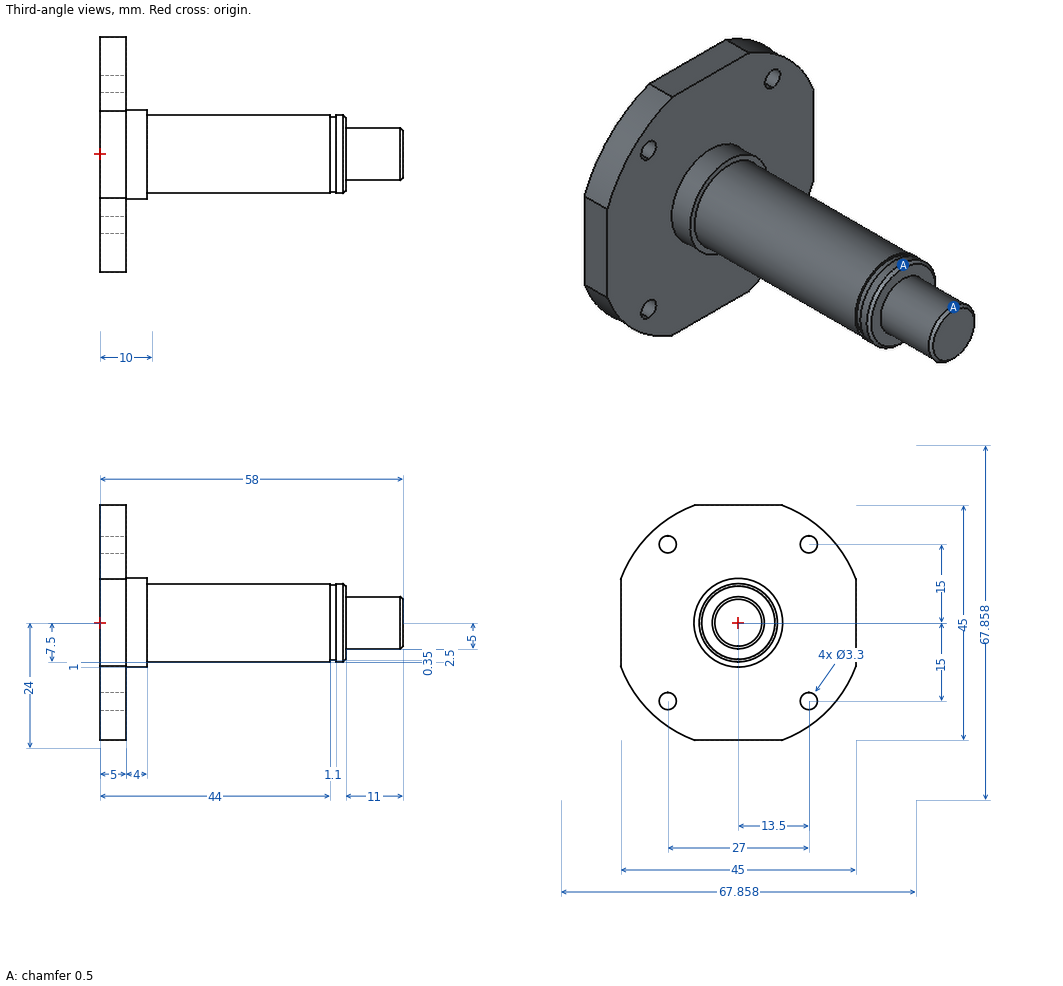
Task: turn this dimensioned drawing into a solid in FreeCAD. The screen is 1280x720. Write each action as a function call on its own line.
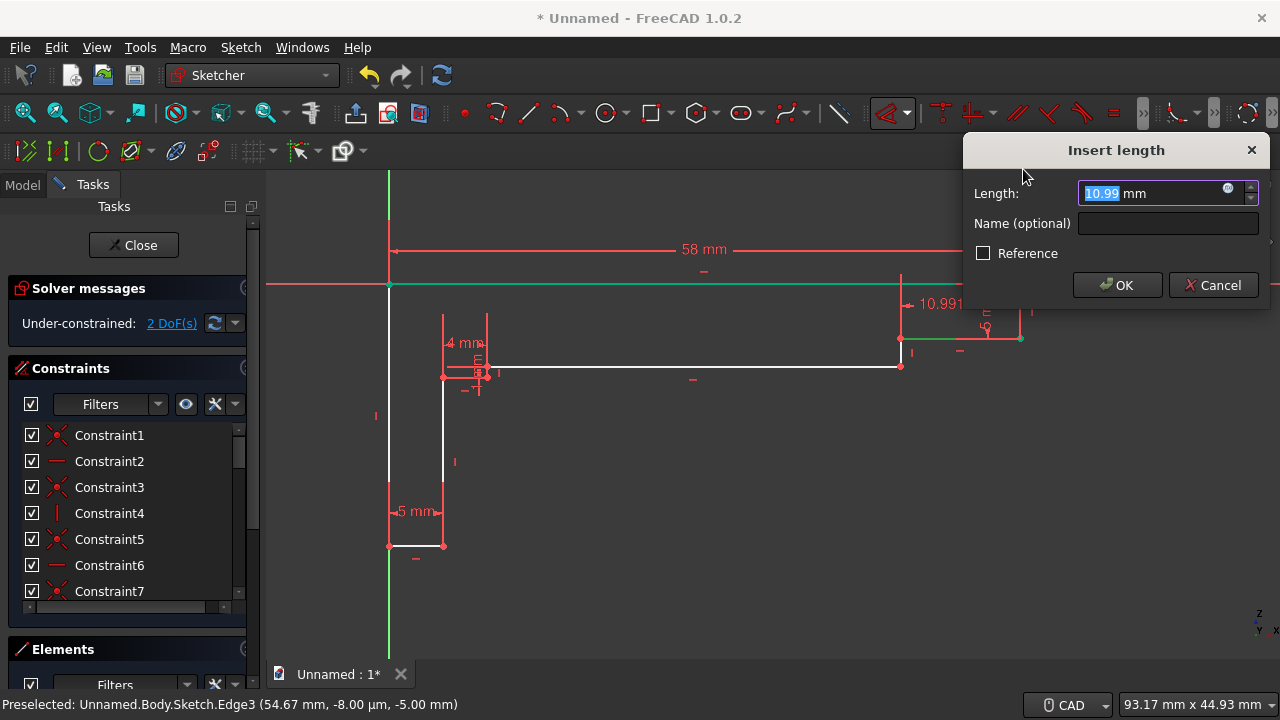
text(11)
key(Return)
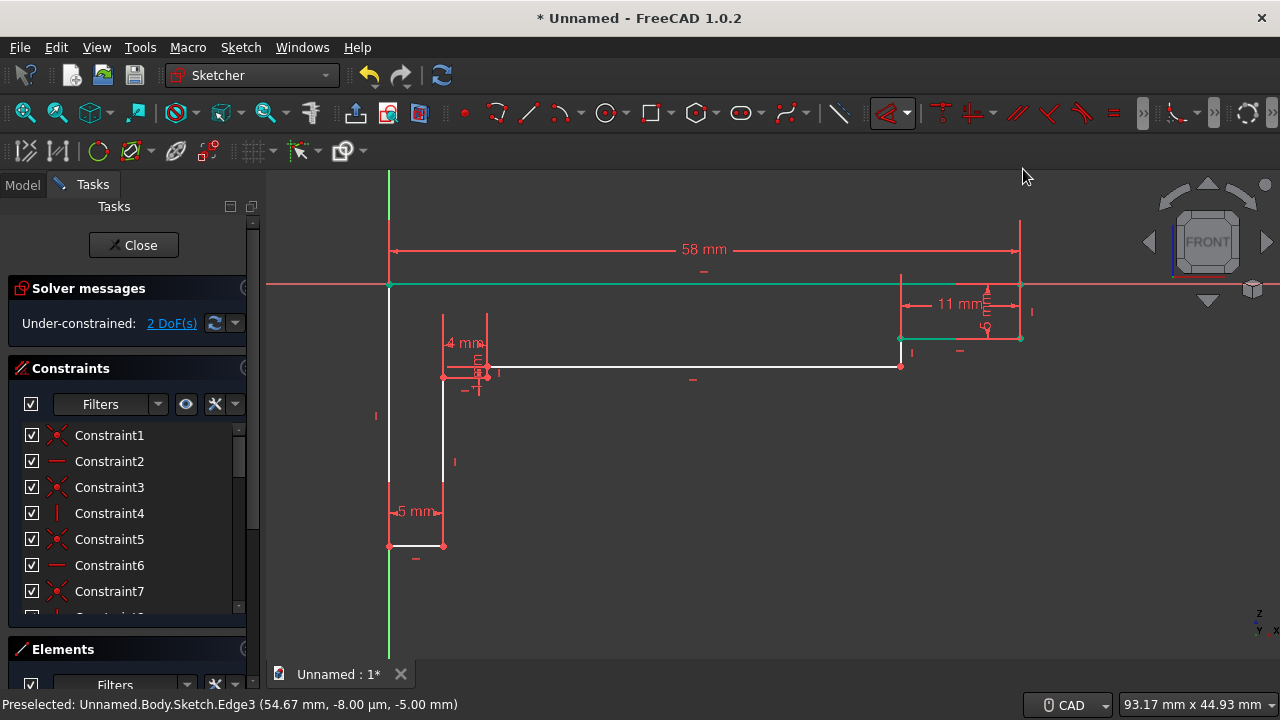
click(389, 467)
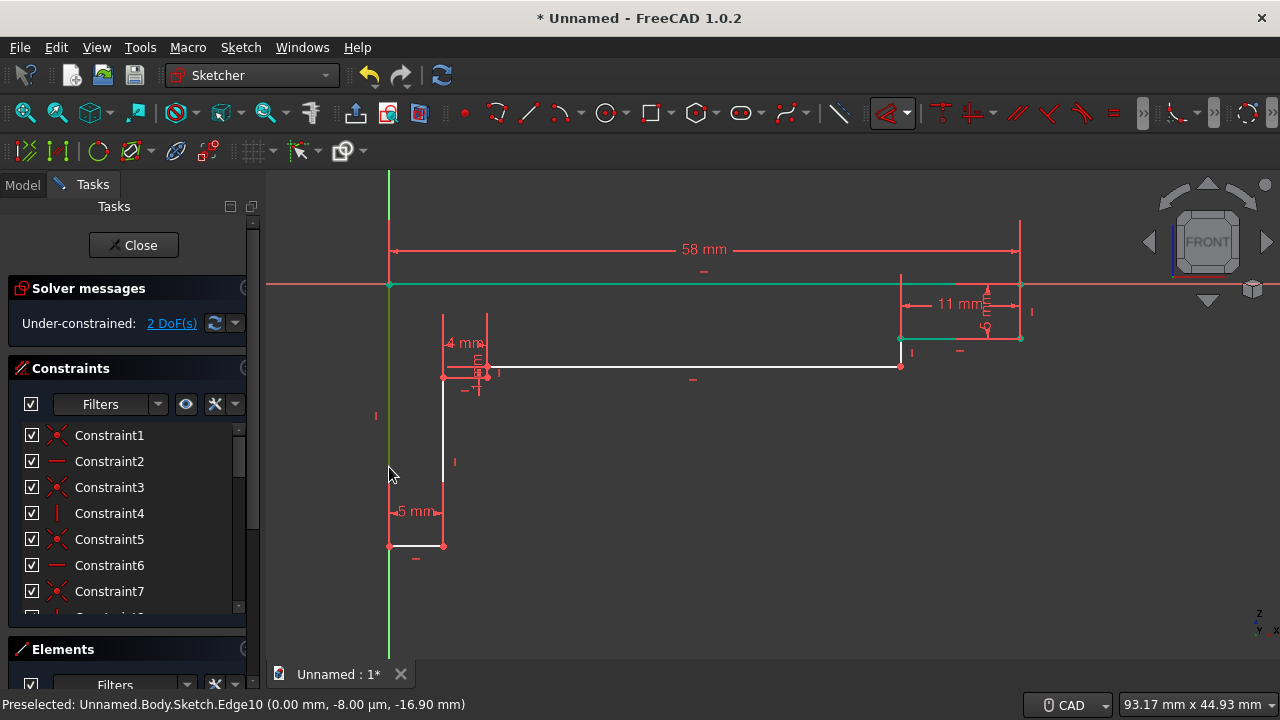
key(i)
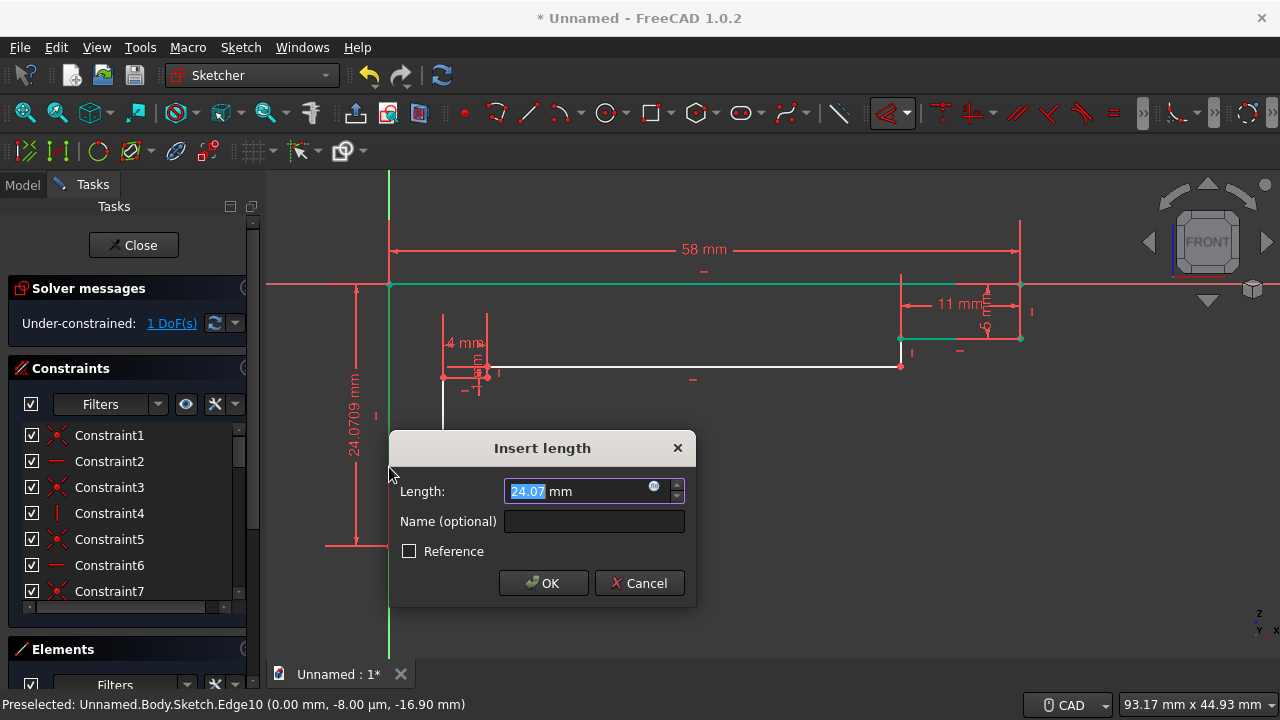
text(24)
key(Return)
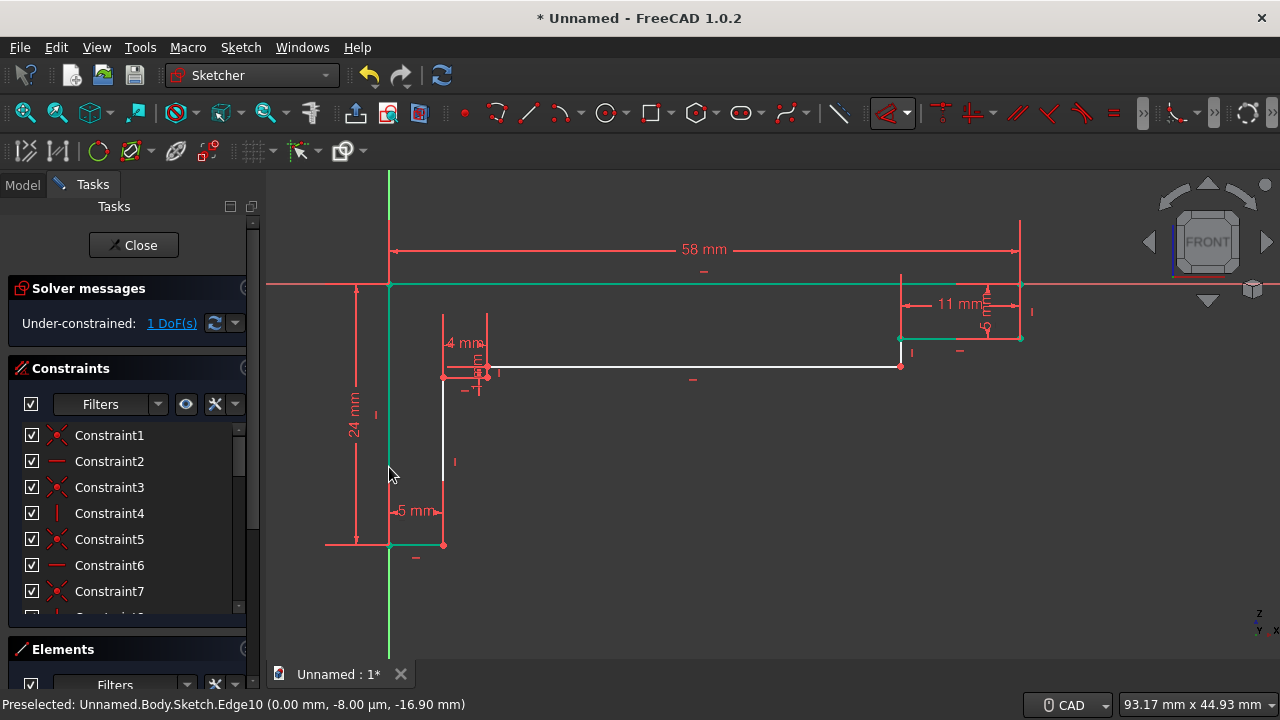
scroll(901, 350, up, 2)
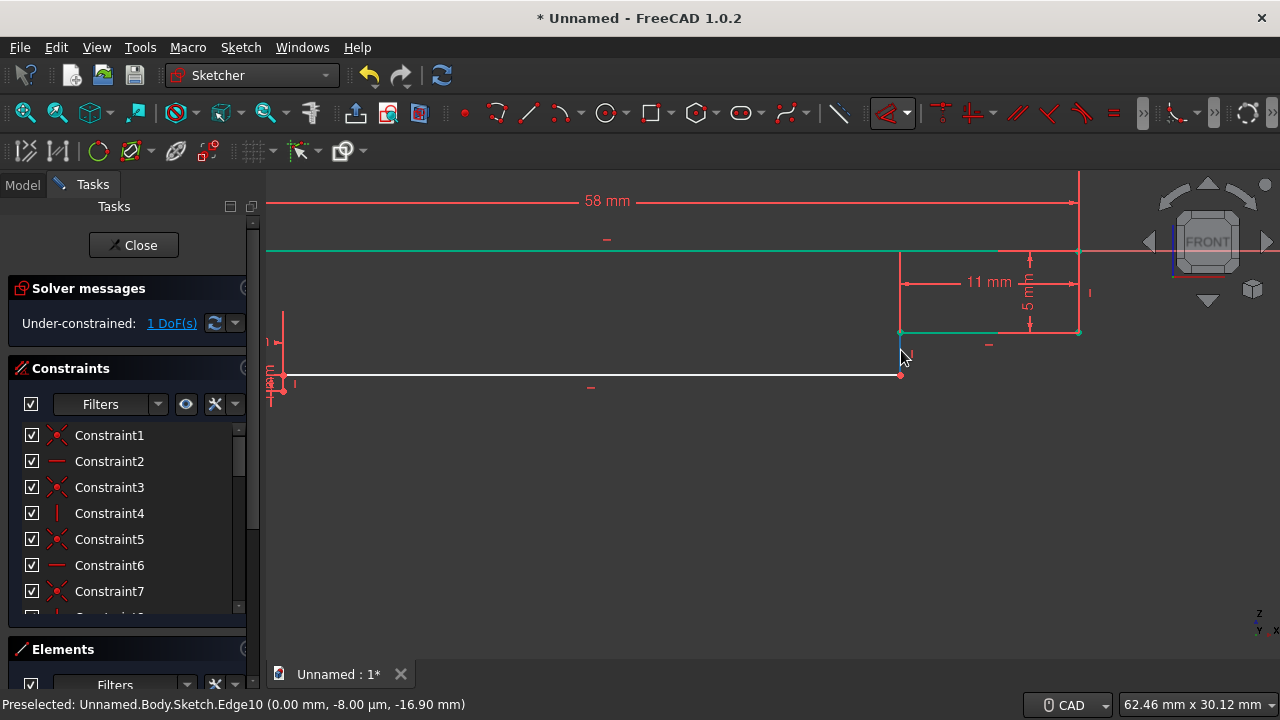
click(900, 350)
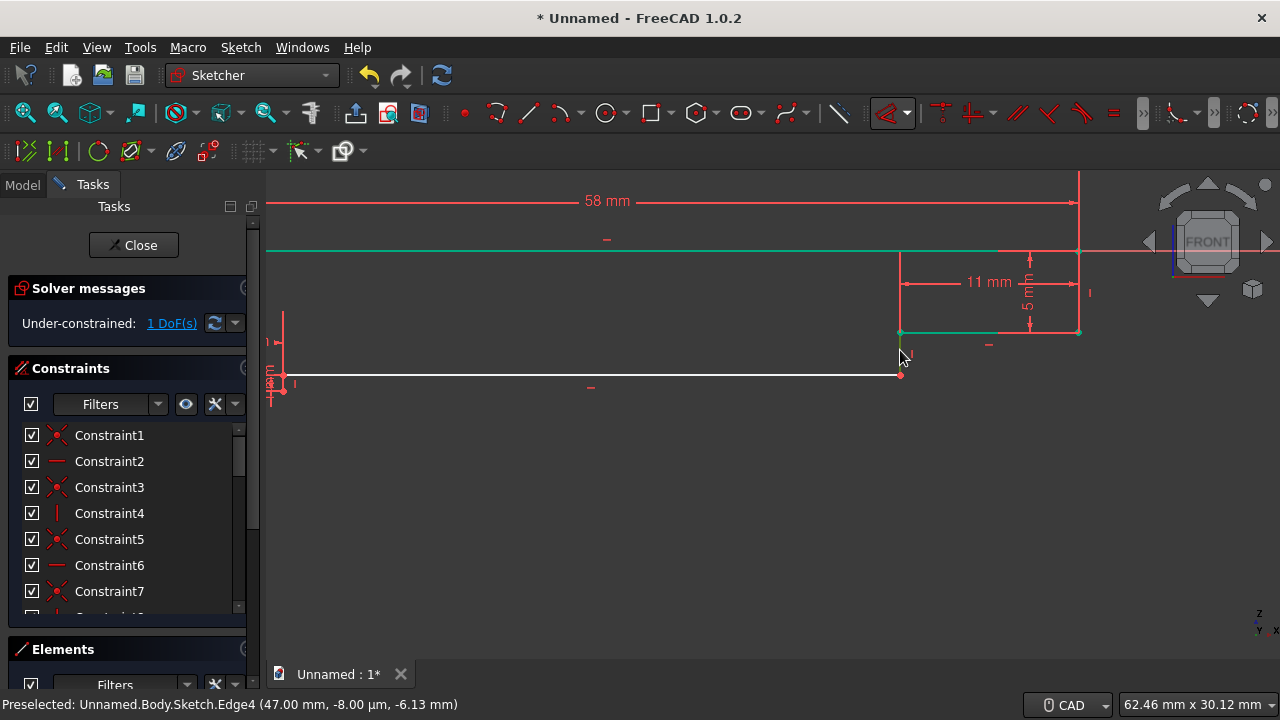
key(i)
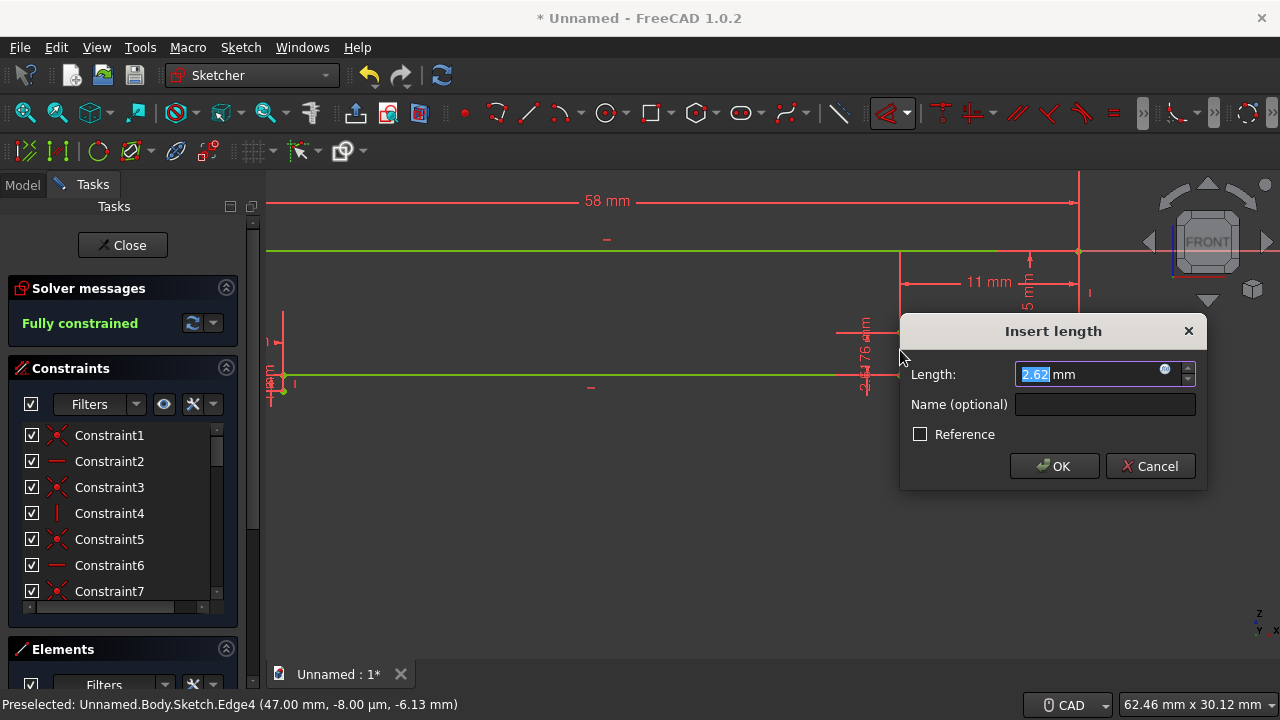
text(2.5)
key(Return)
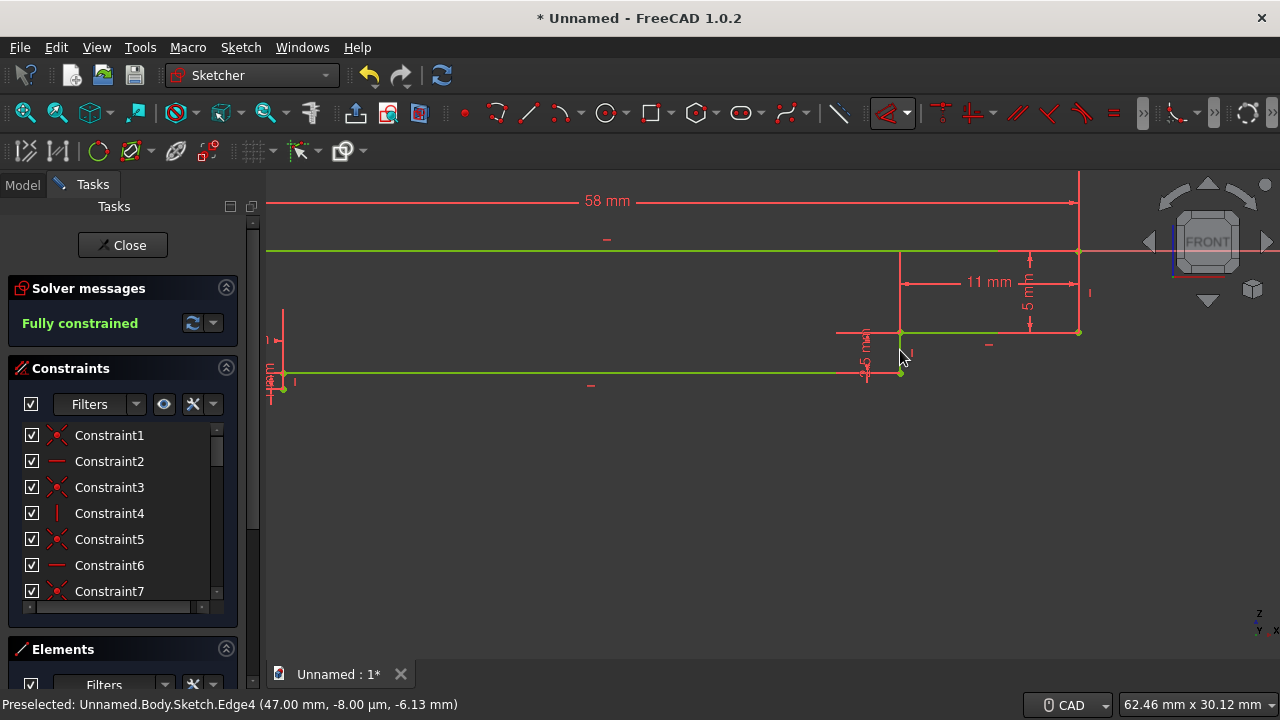
click(123, 245)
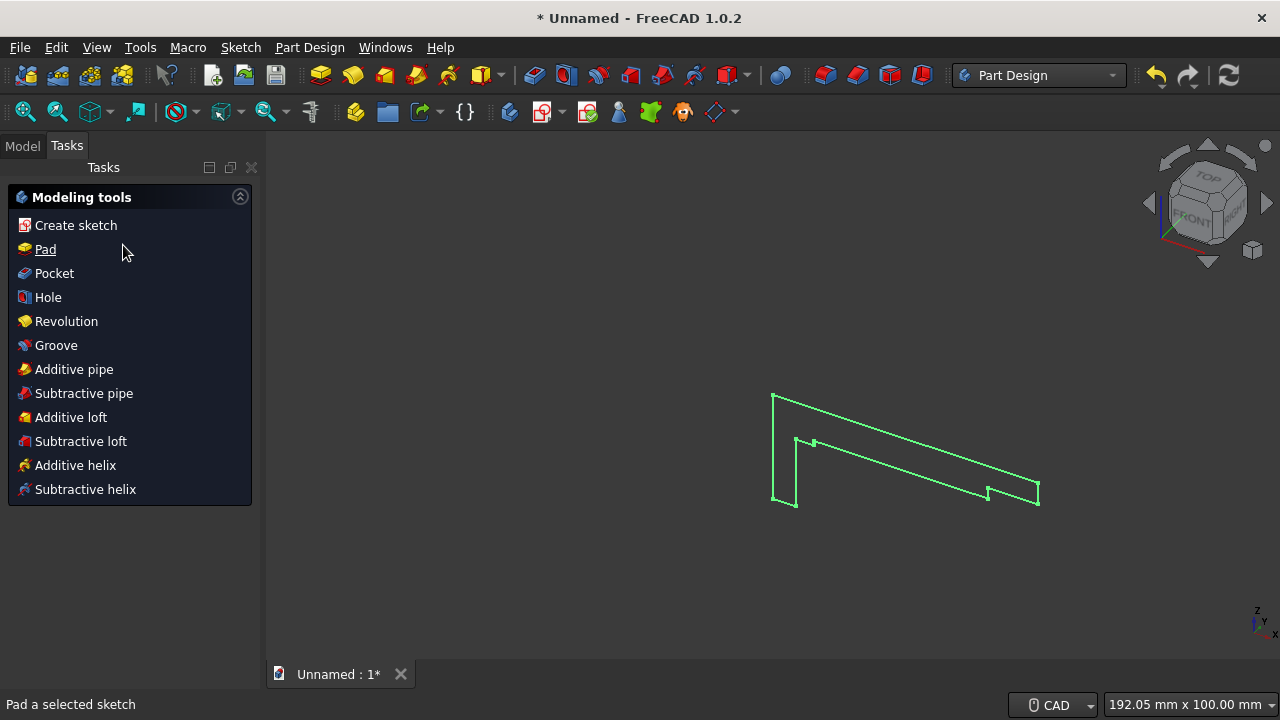
click(354, 76)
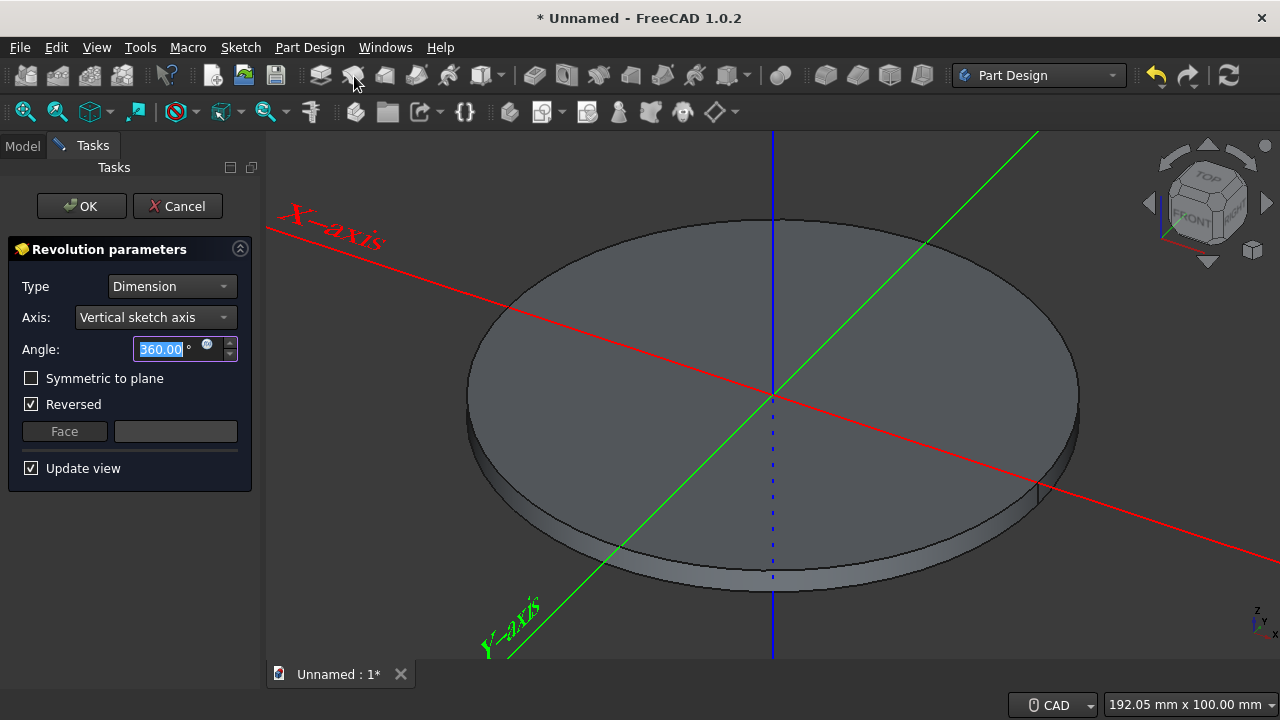
click(156, 318)